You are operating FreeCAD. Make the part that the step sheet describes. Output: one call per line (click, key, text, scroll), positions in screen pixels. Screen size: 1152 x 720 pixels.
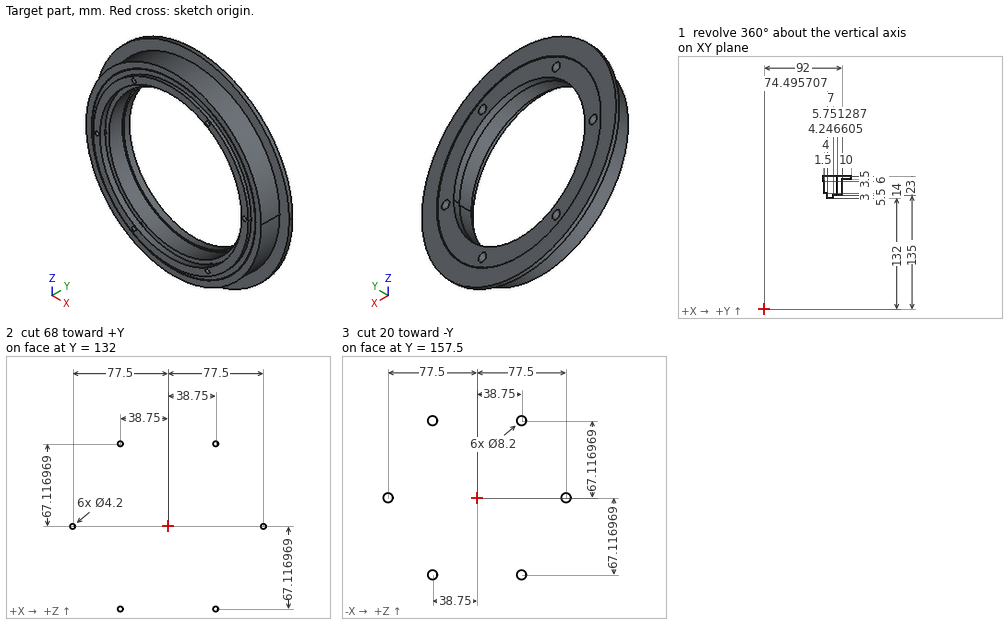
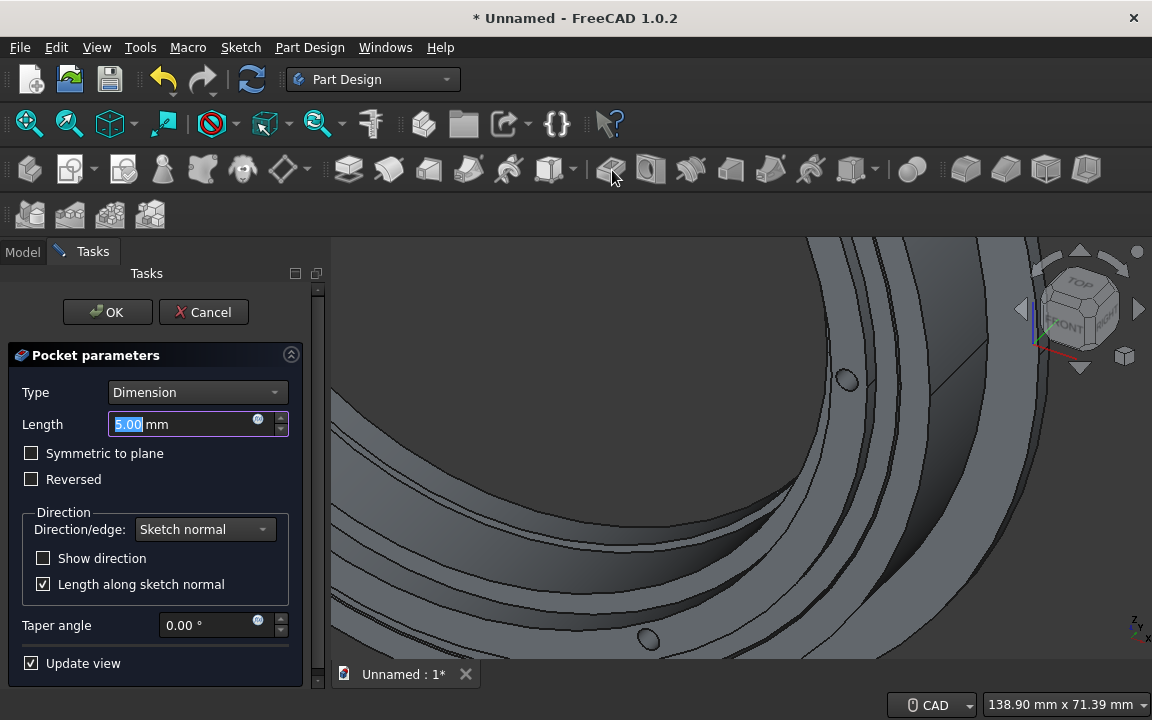
text(68)
key(Tab)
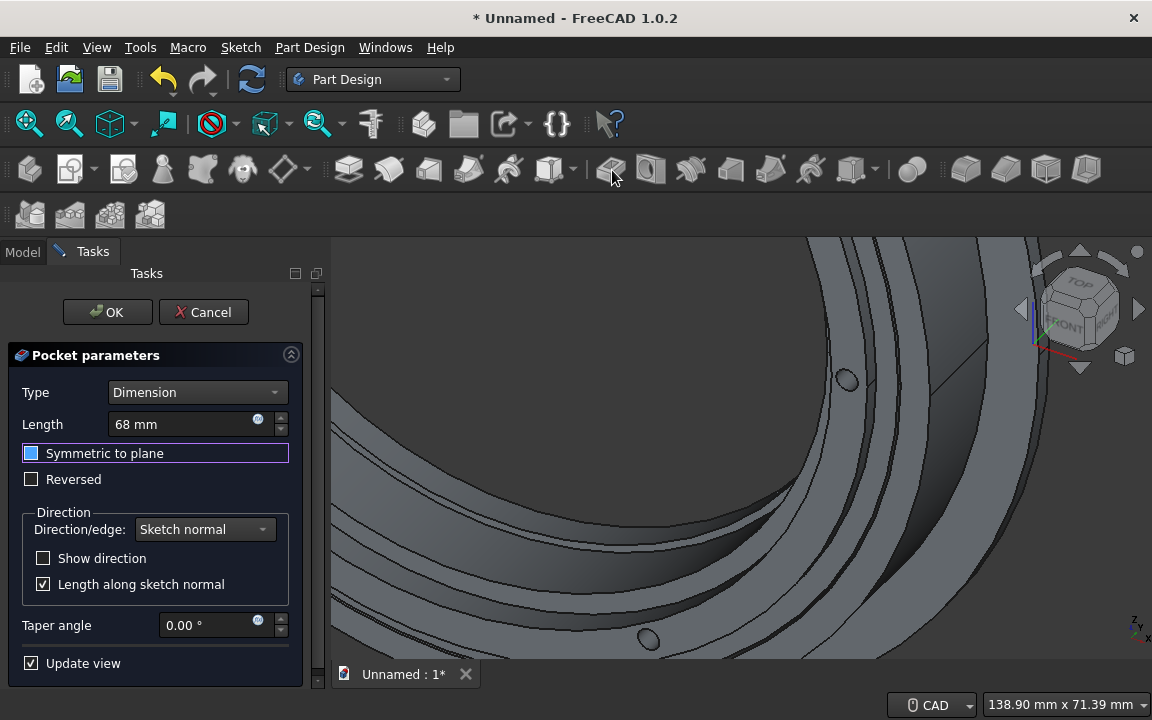
click(108, 312)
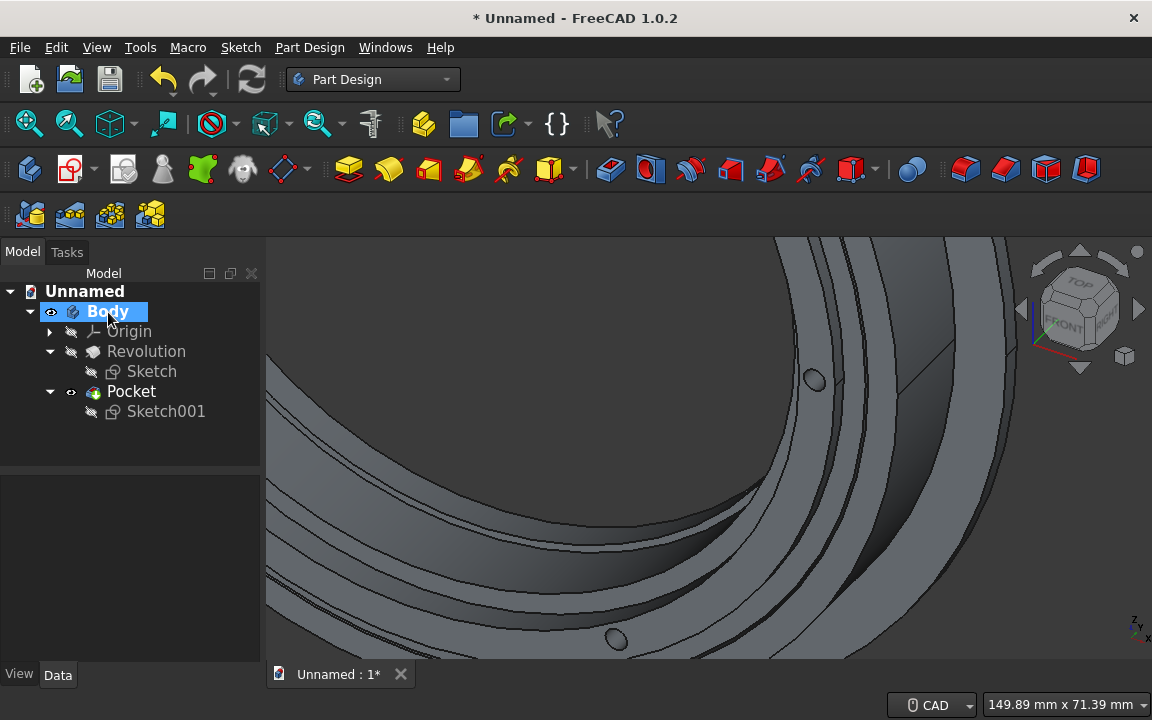
click(30, 124)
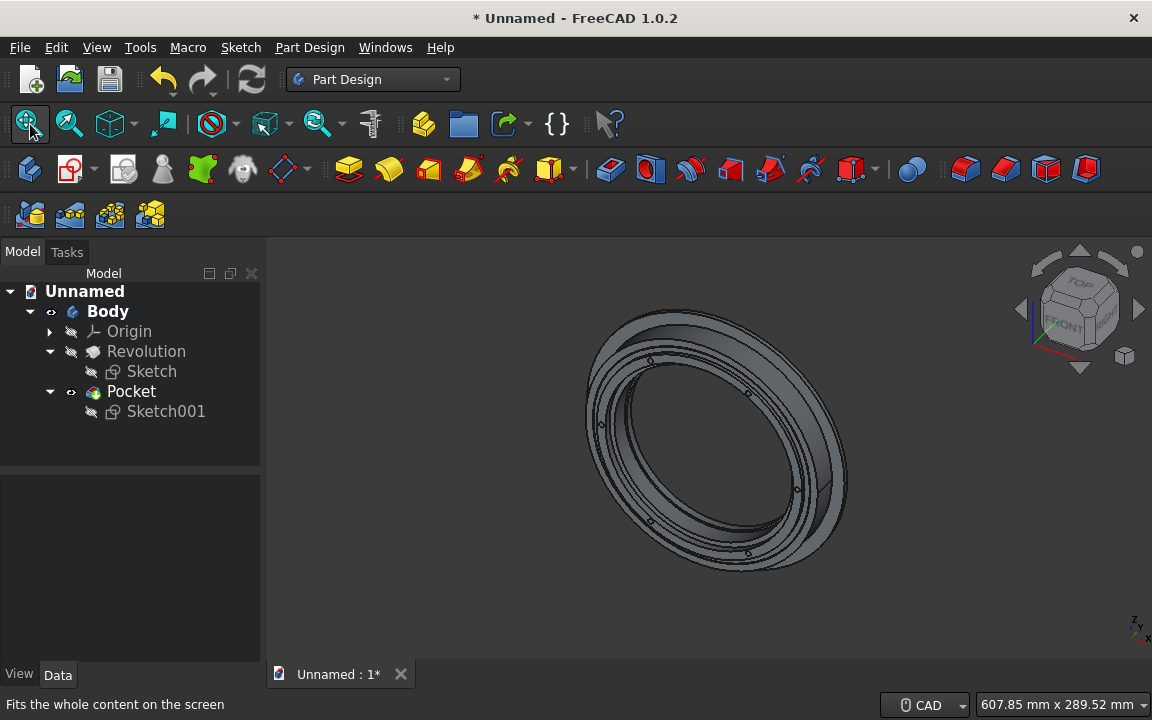
key(4)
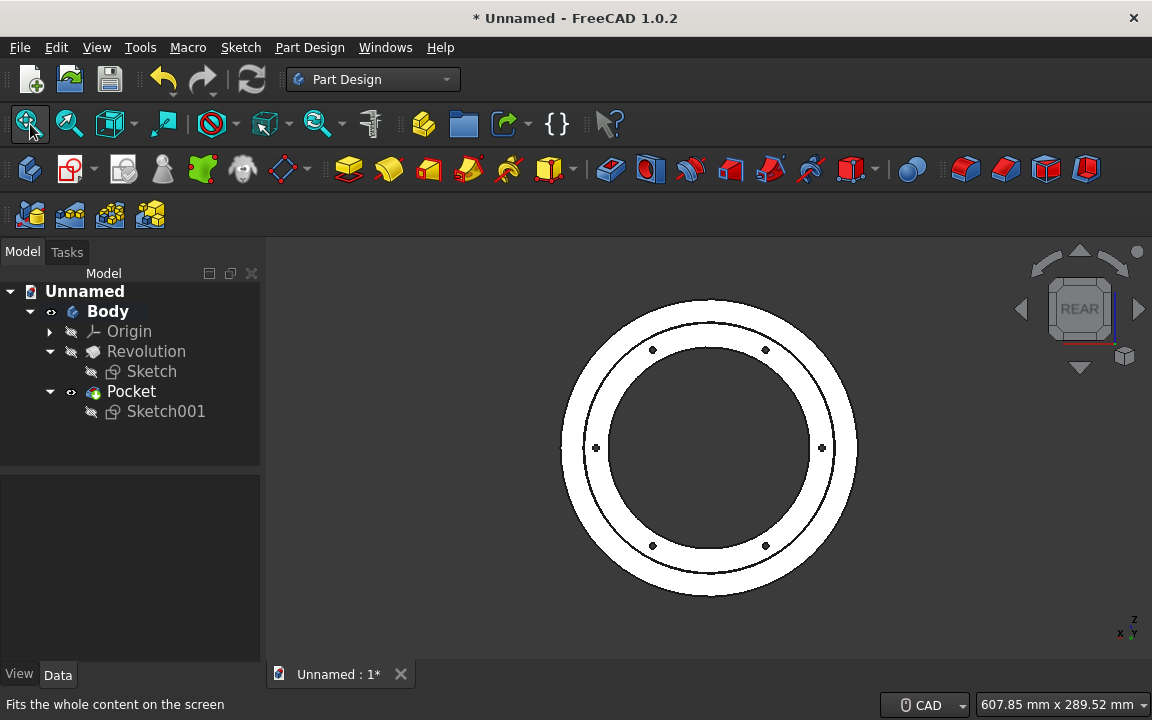
click(602, 483)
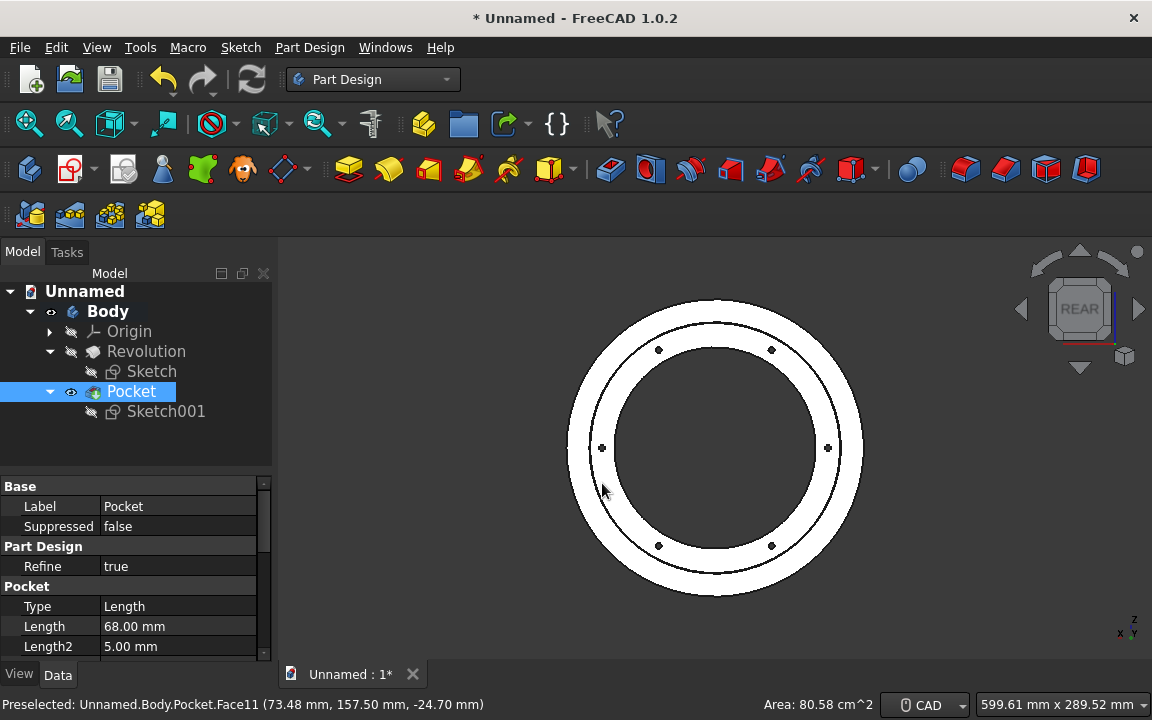
click(70, 170)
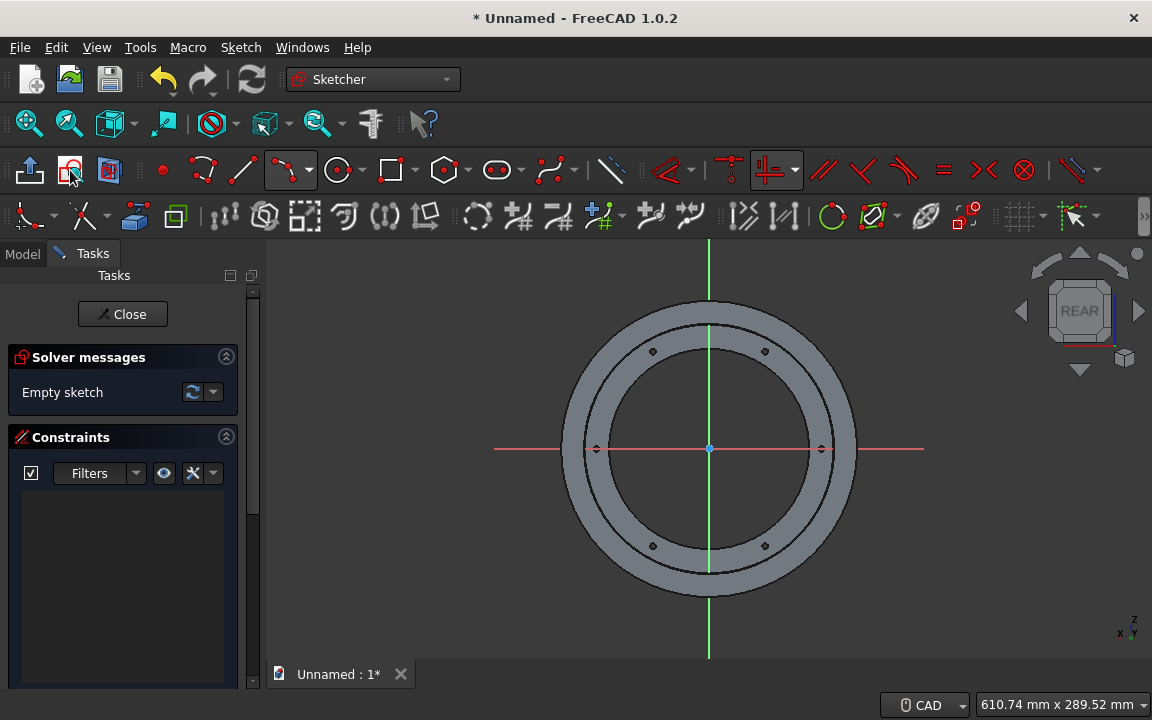
click(110, 170)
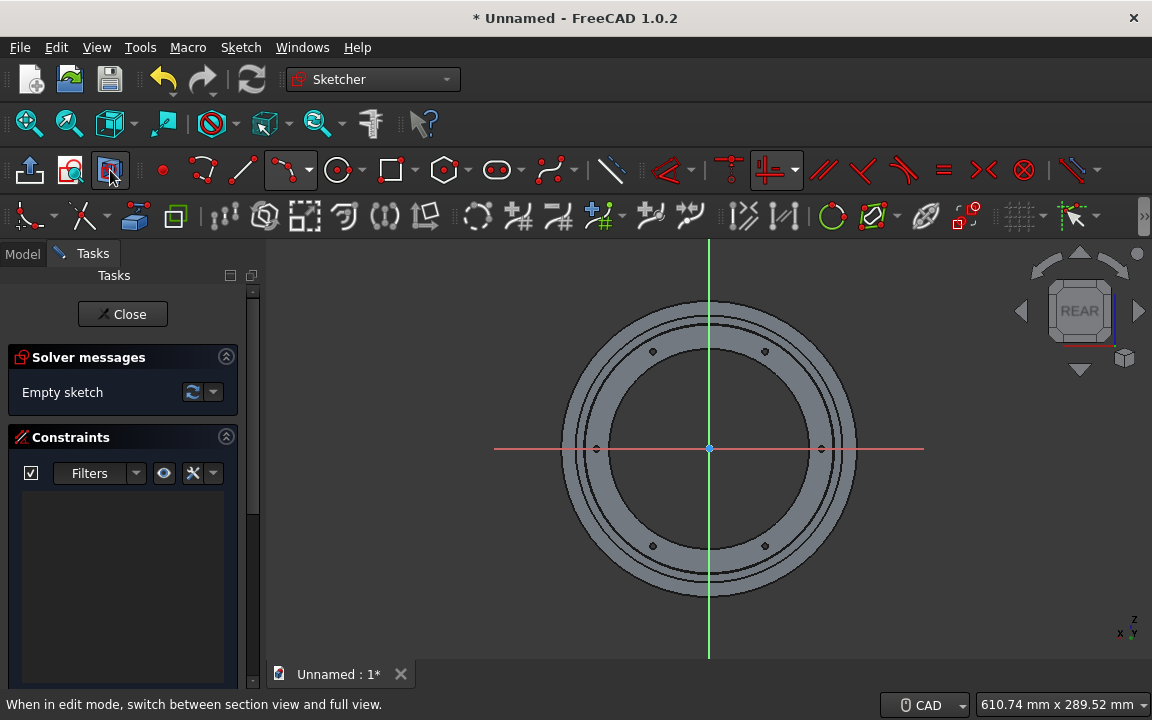
click(338, 170)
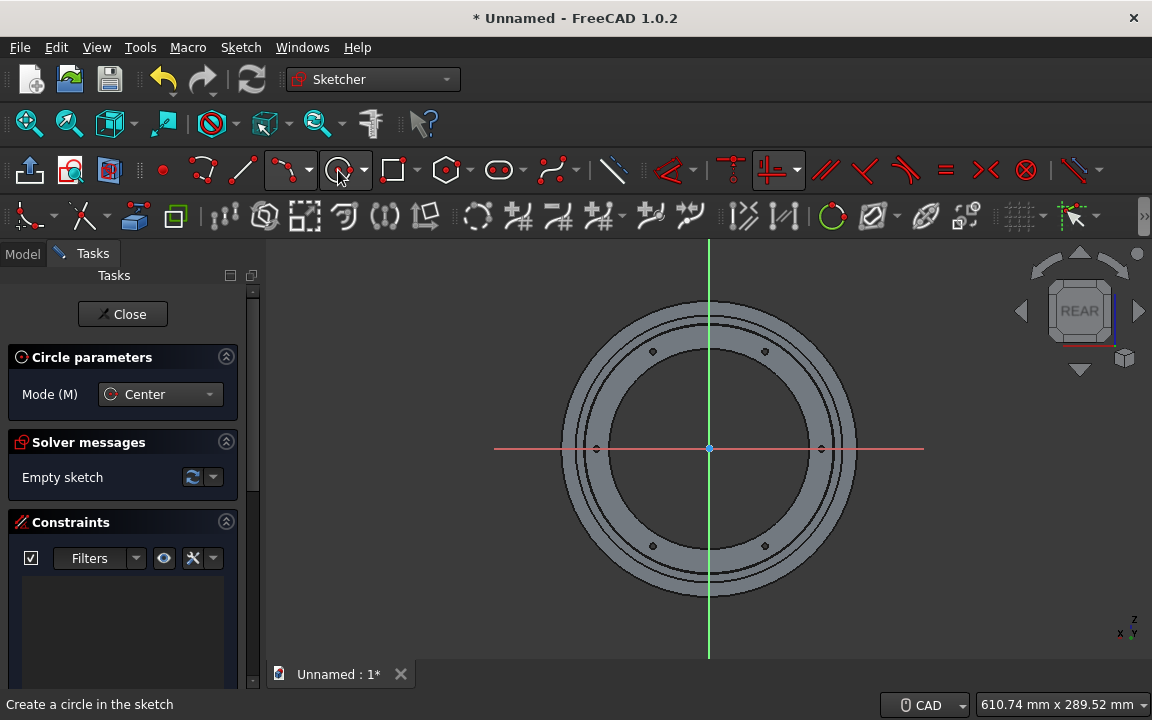
scroll(765, 352, up, 7)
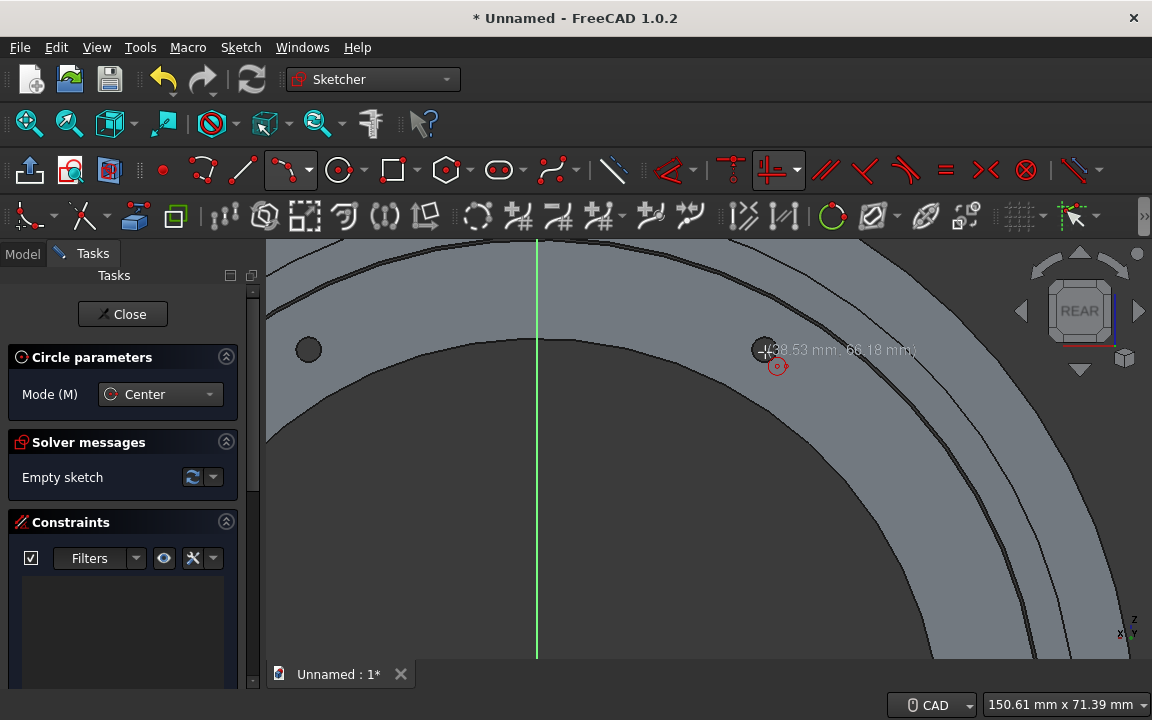
scroll(685, 322, down, 6)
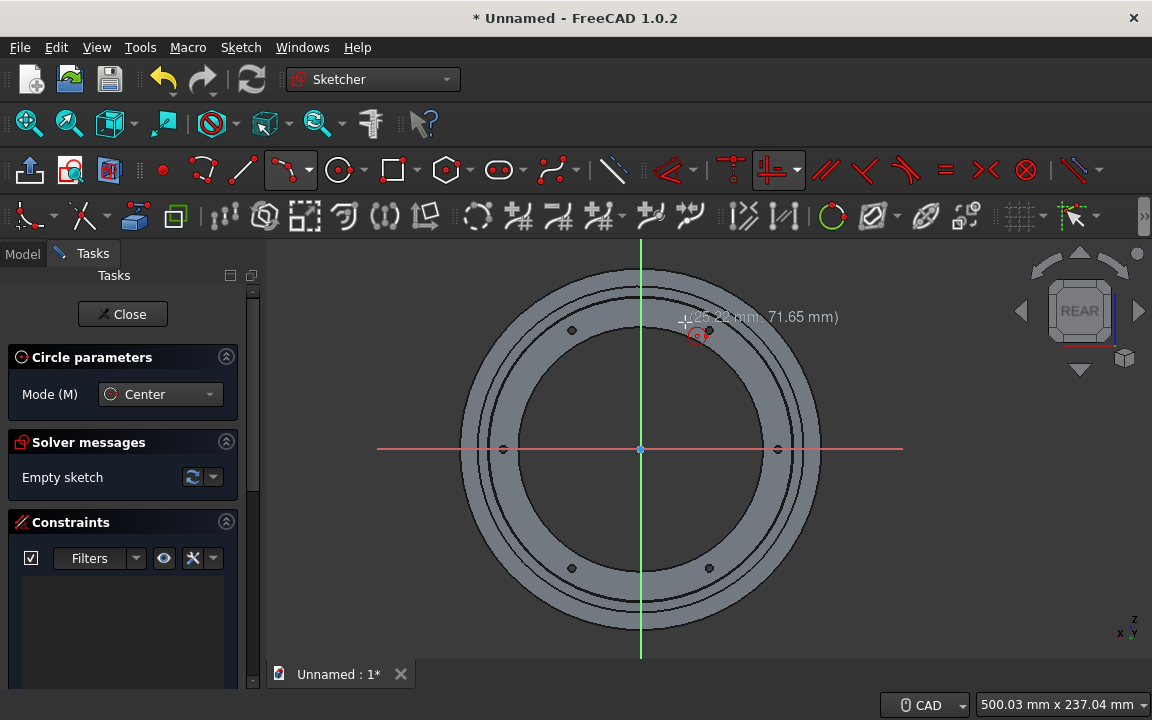
click(709, 330)
move(714, 325)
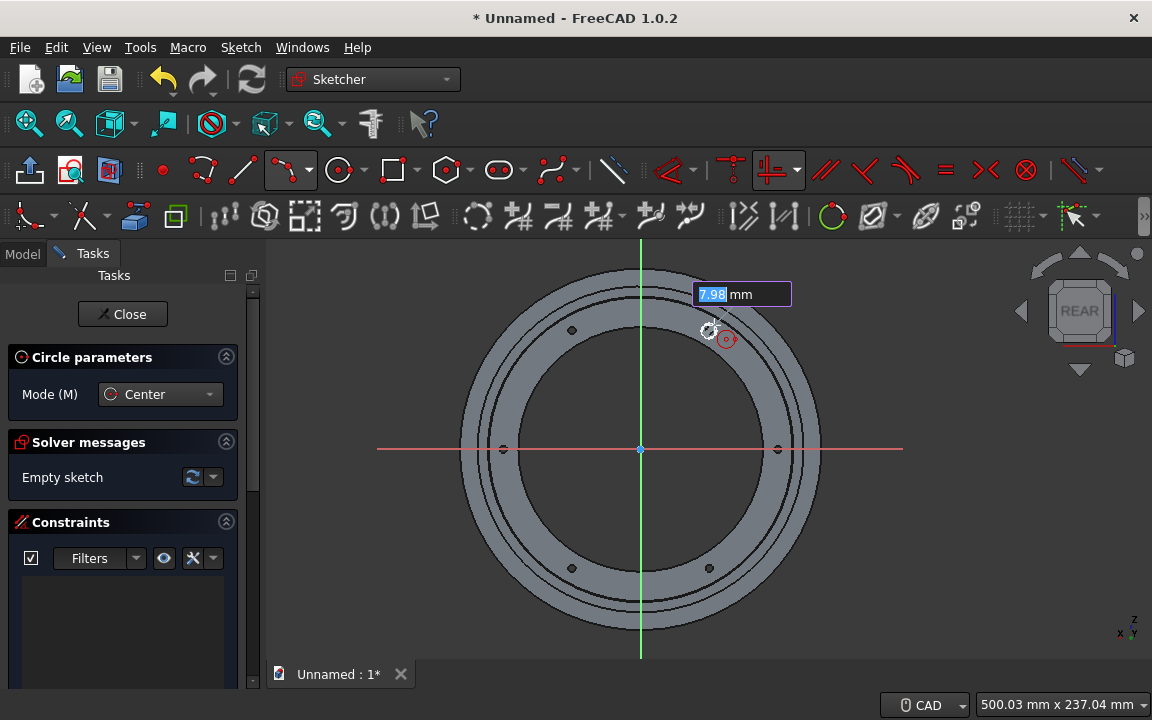
text(8.2)
key(Return)